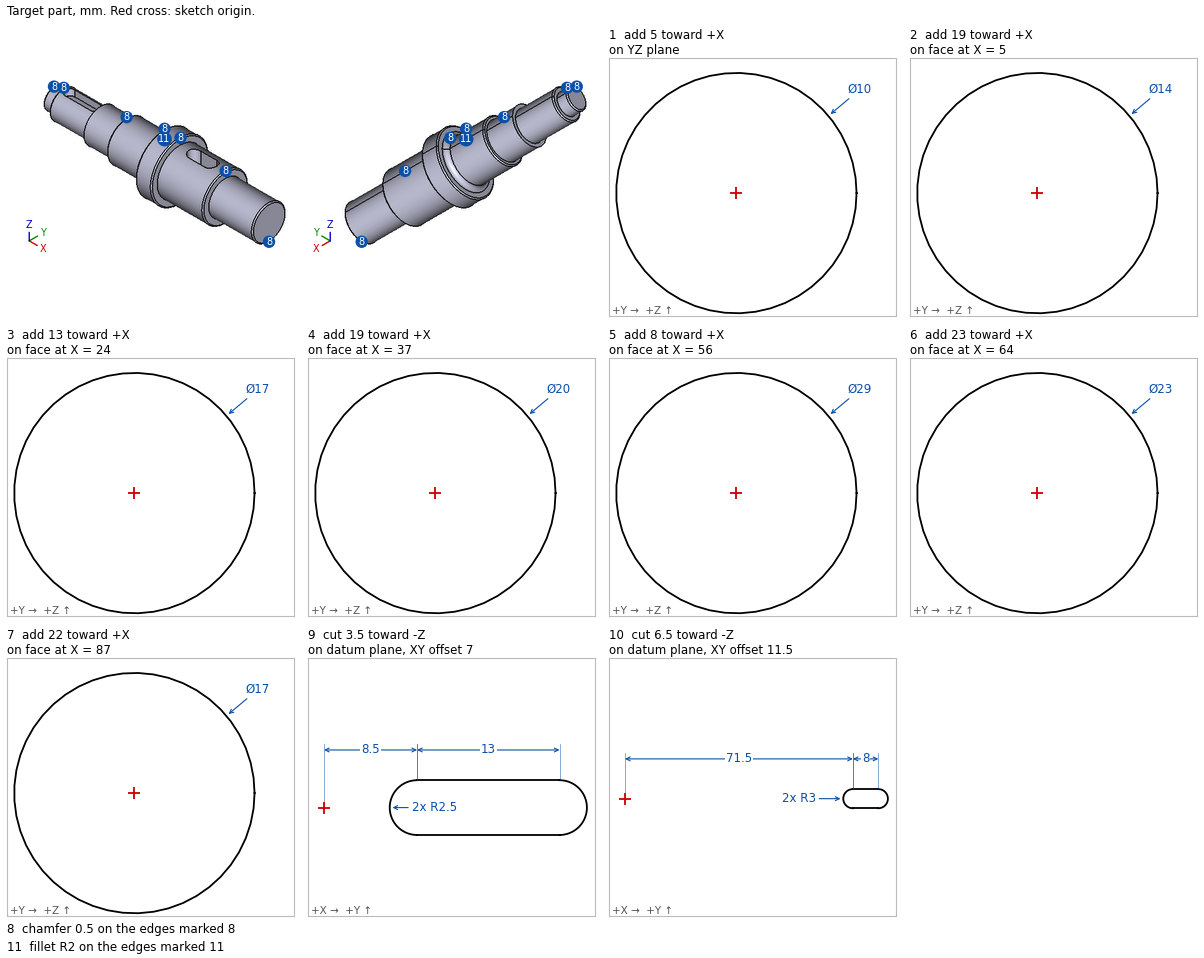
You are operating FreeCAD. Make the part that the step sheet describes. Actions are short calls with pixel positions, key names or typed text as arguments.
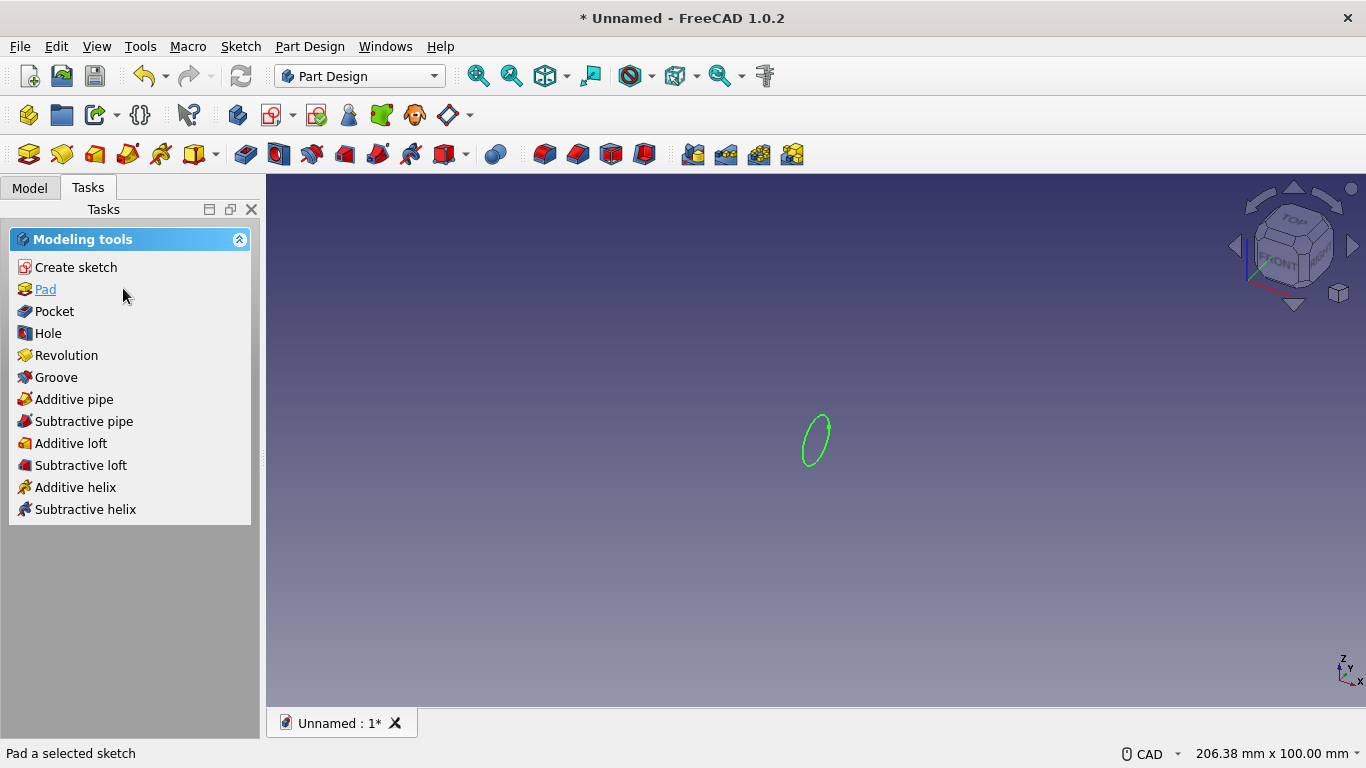
click(29, 154)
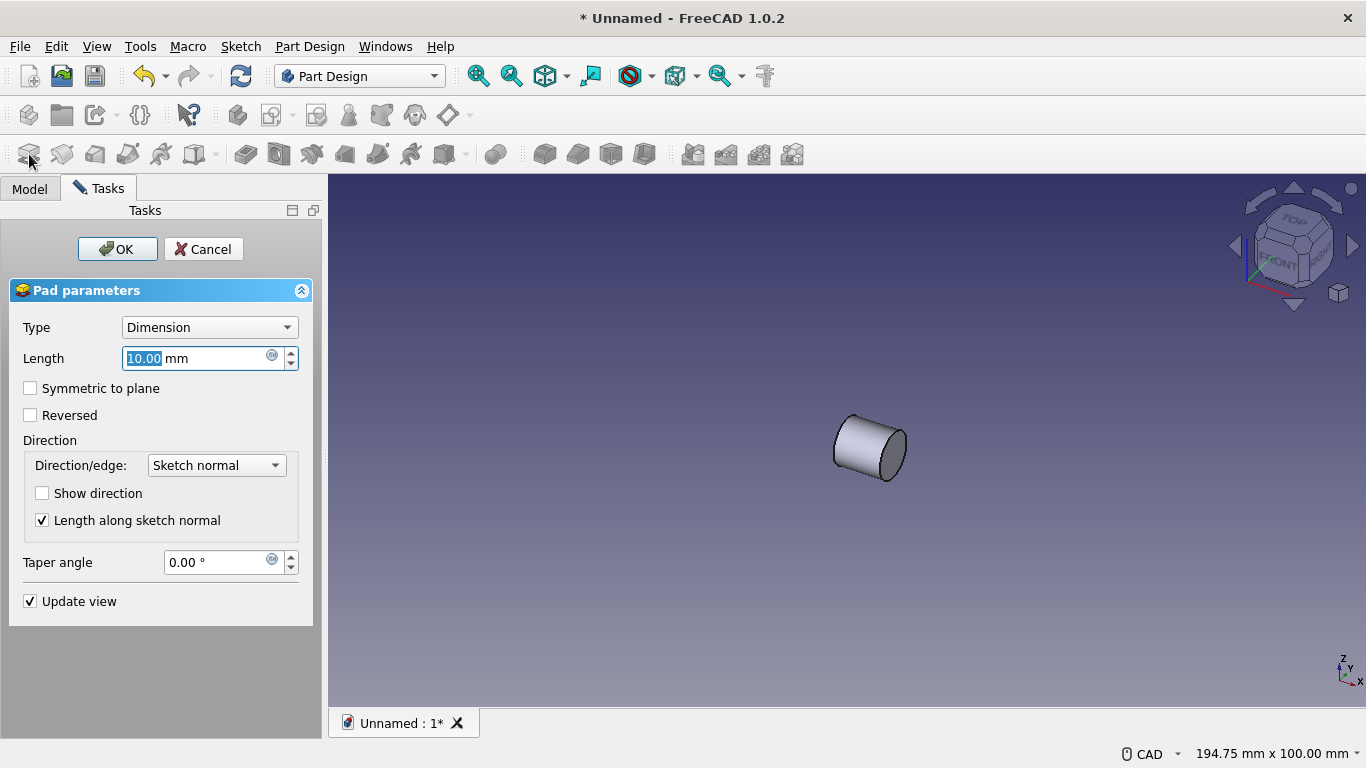
text(5)
key(Tab)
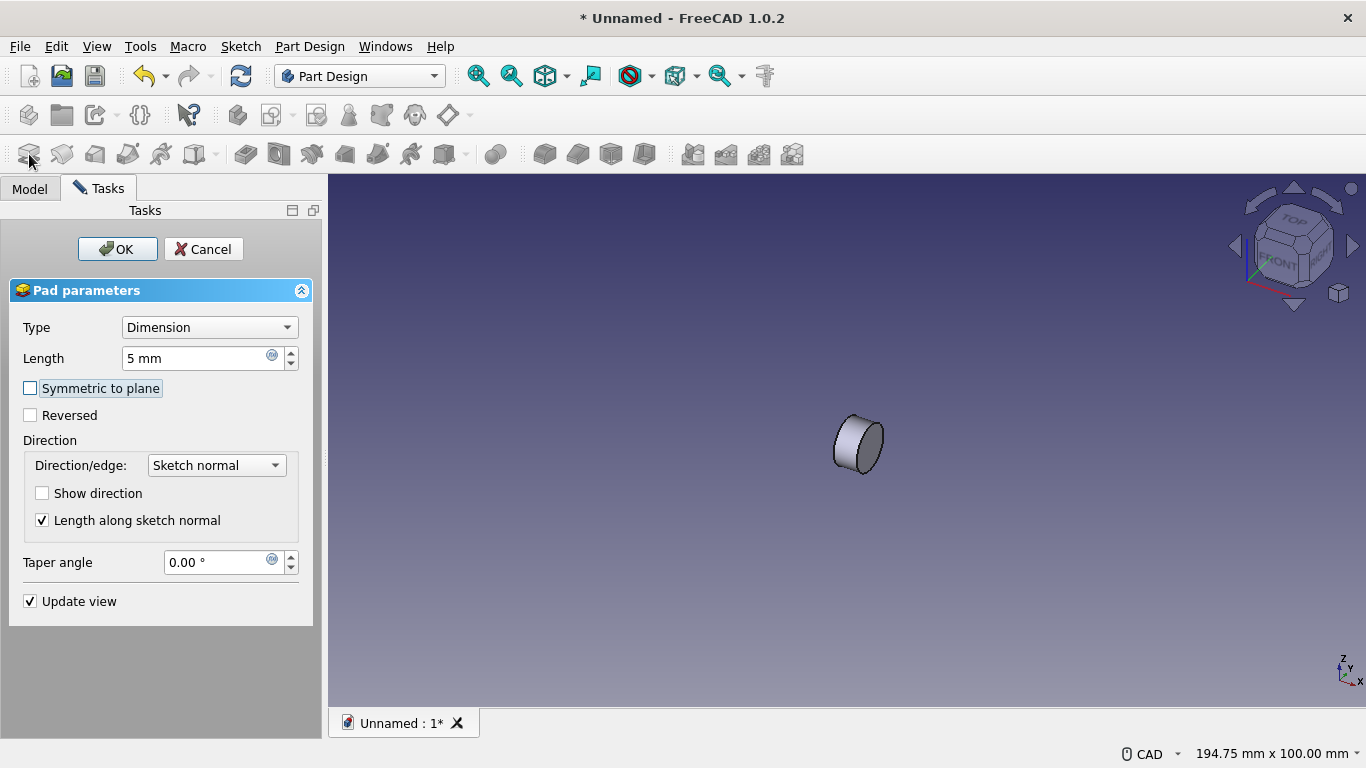
click(118, 249)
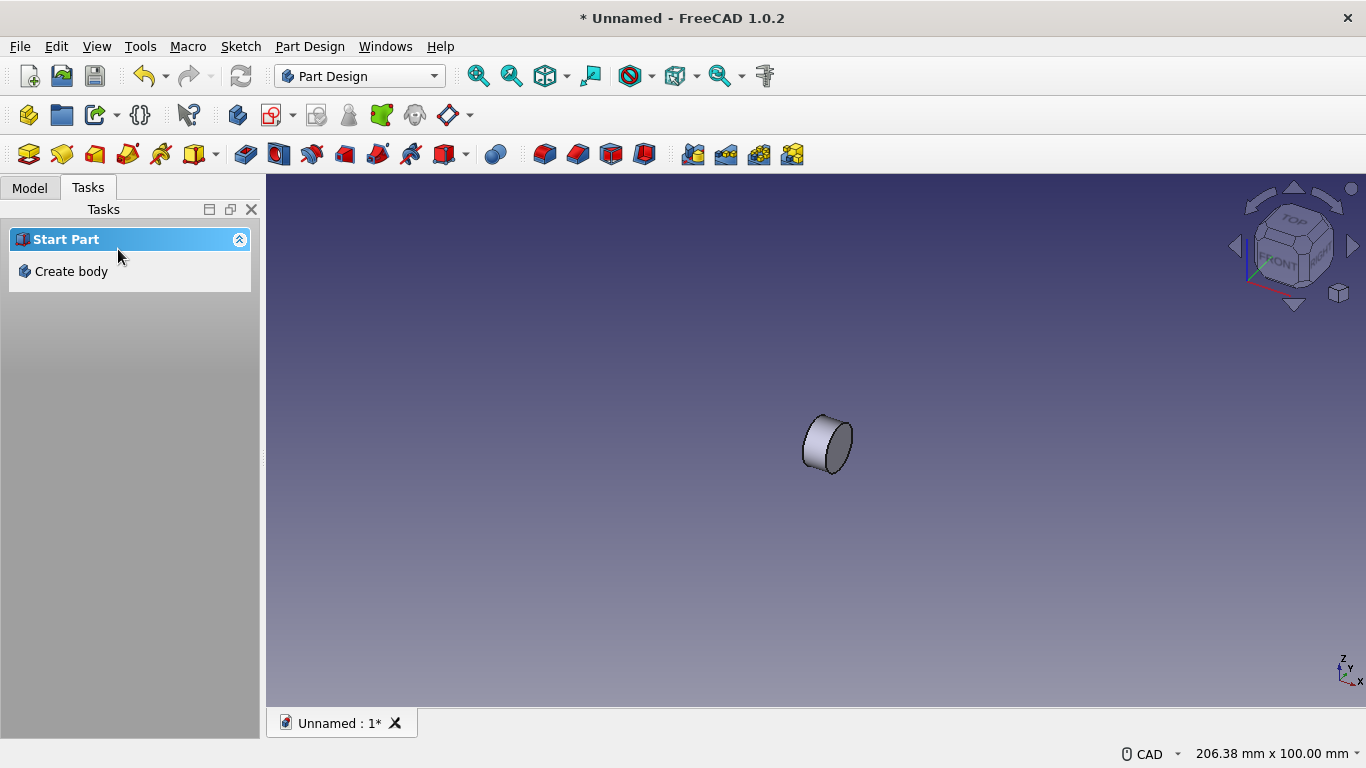
key(v)
key(f)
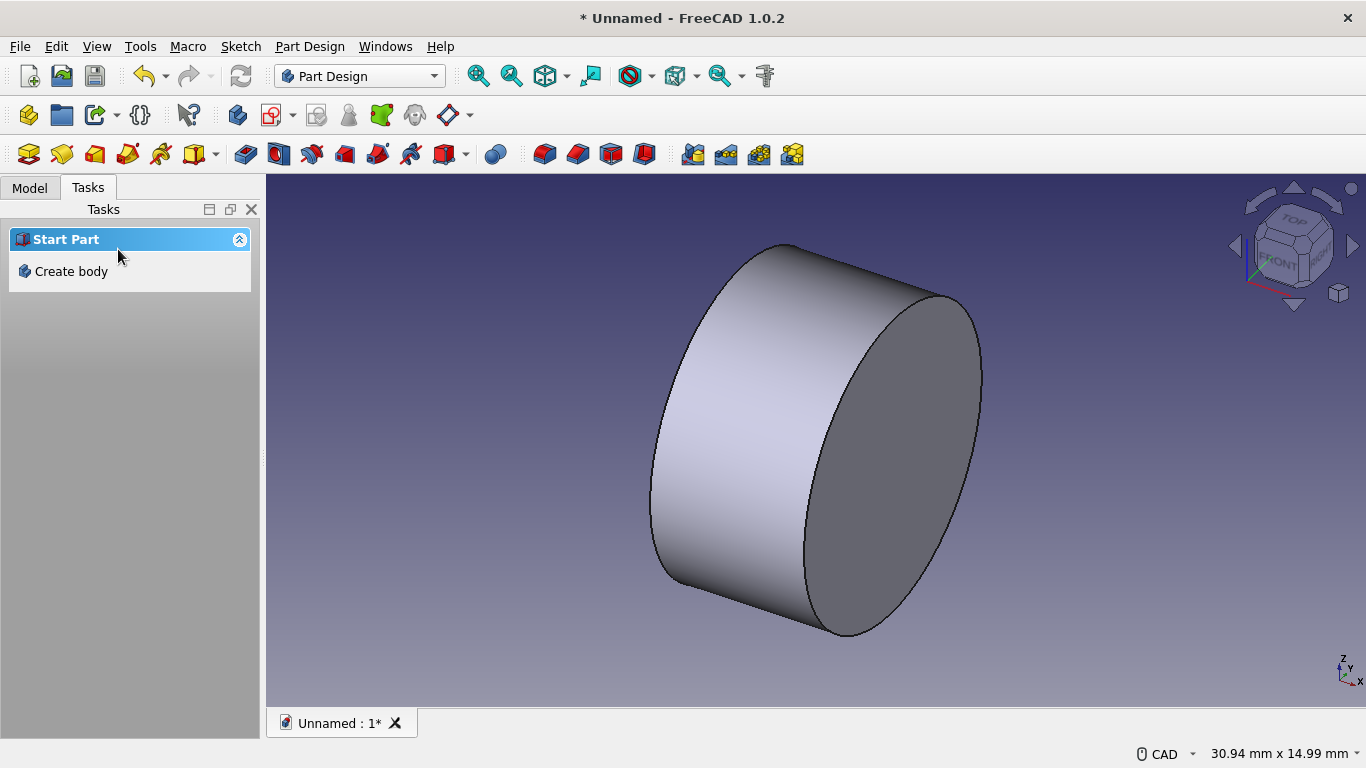
click(893, 465)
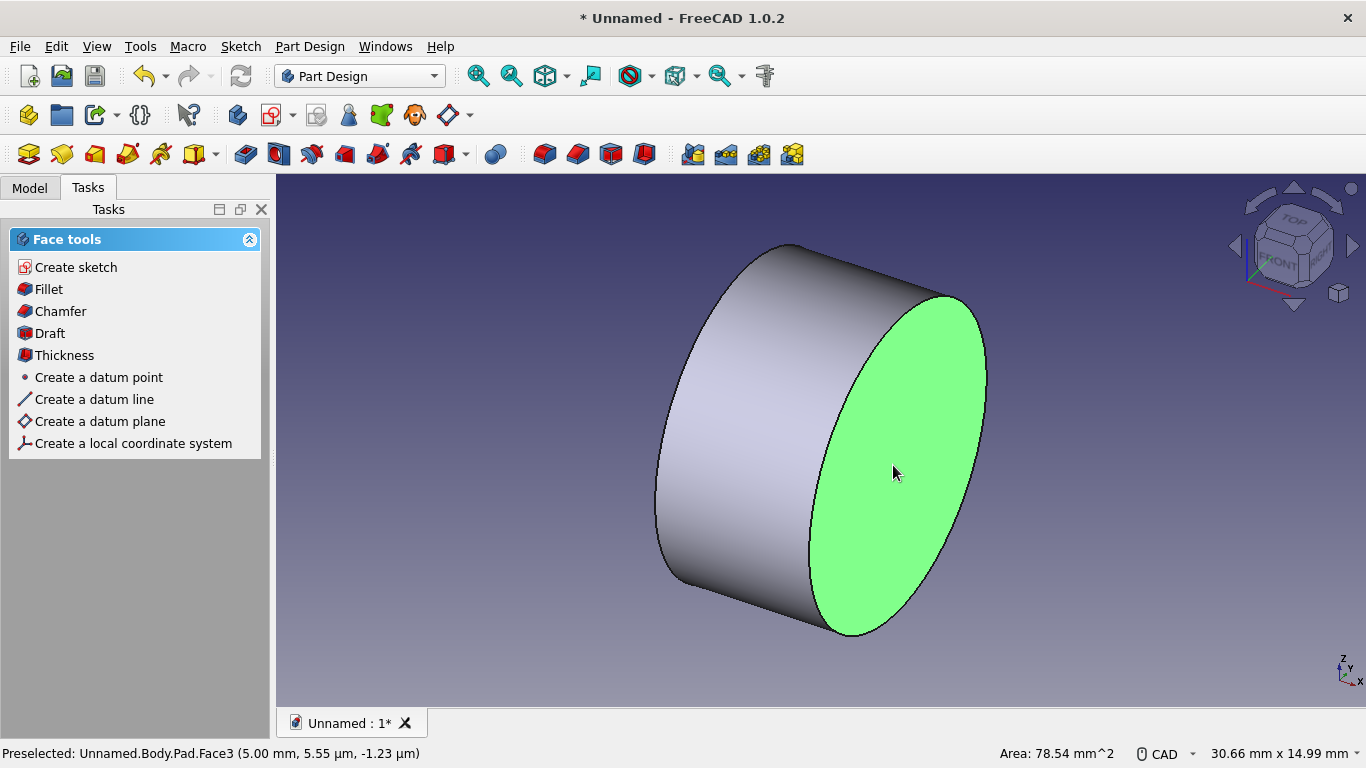
click(270, 116)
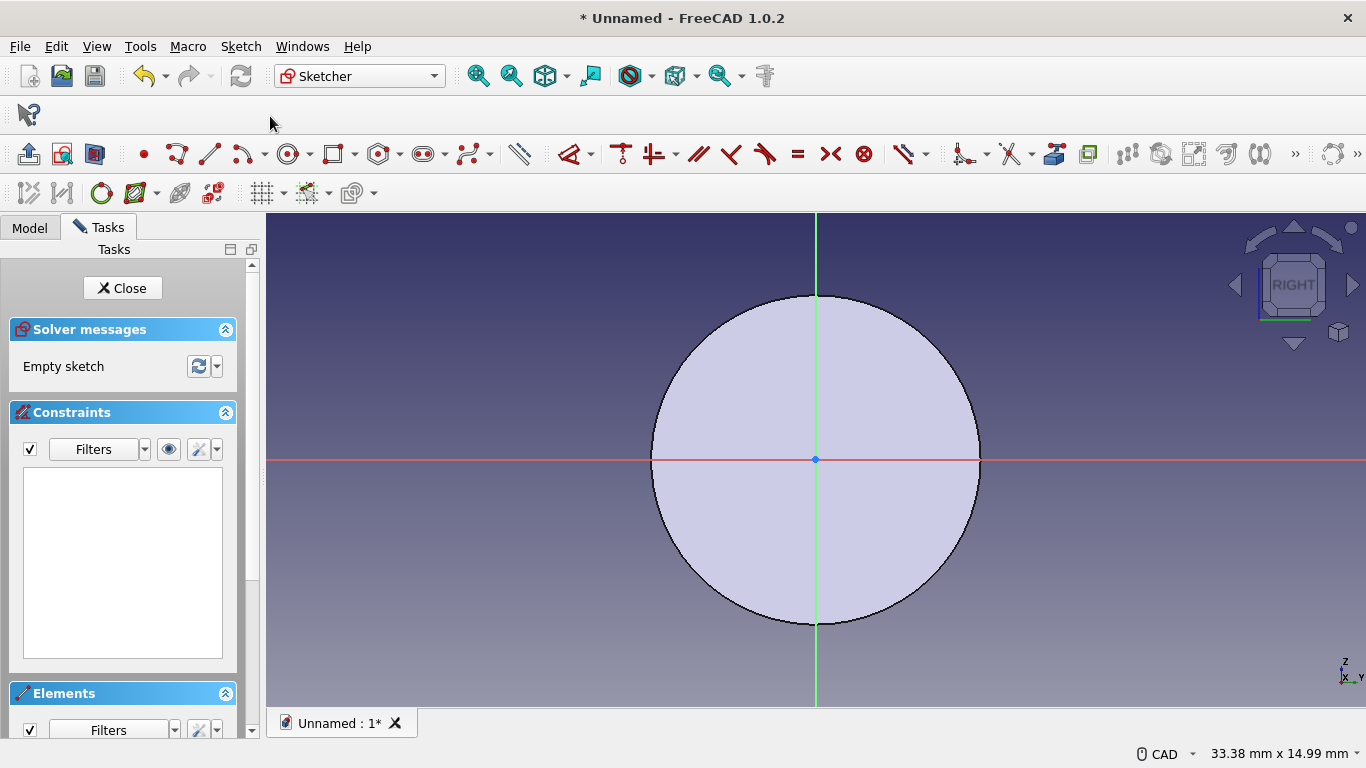
scroll(608, 460, down, 2)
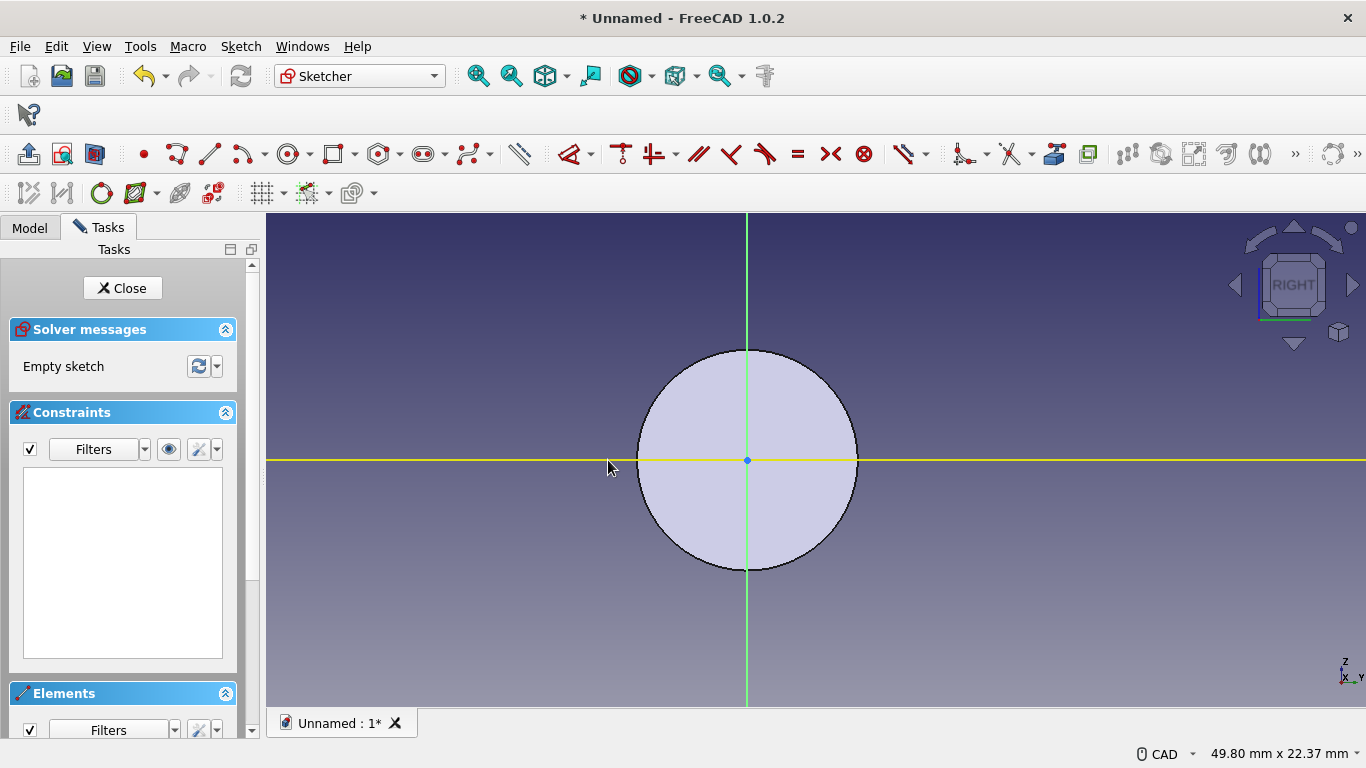
click(288, 154)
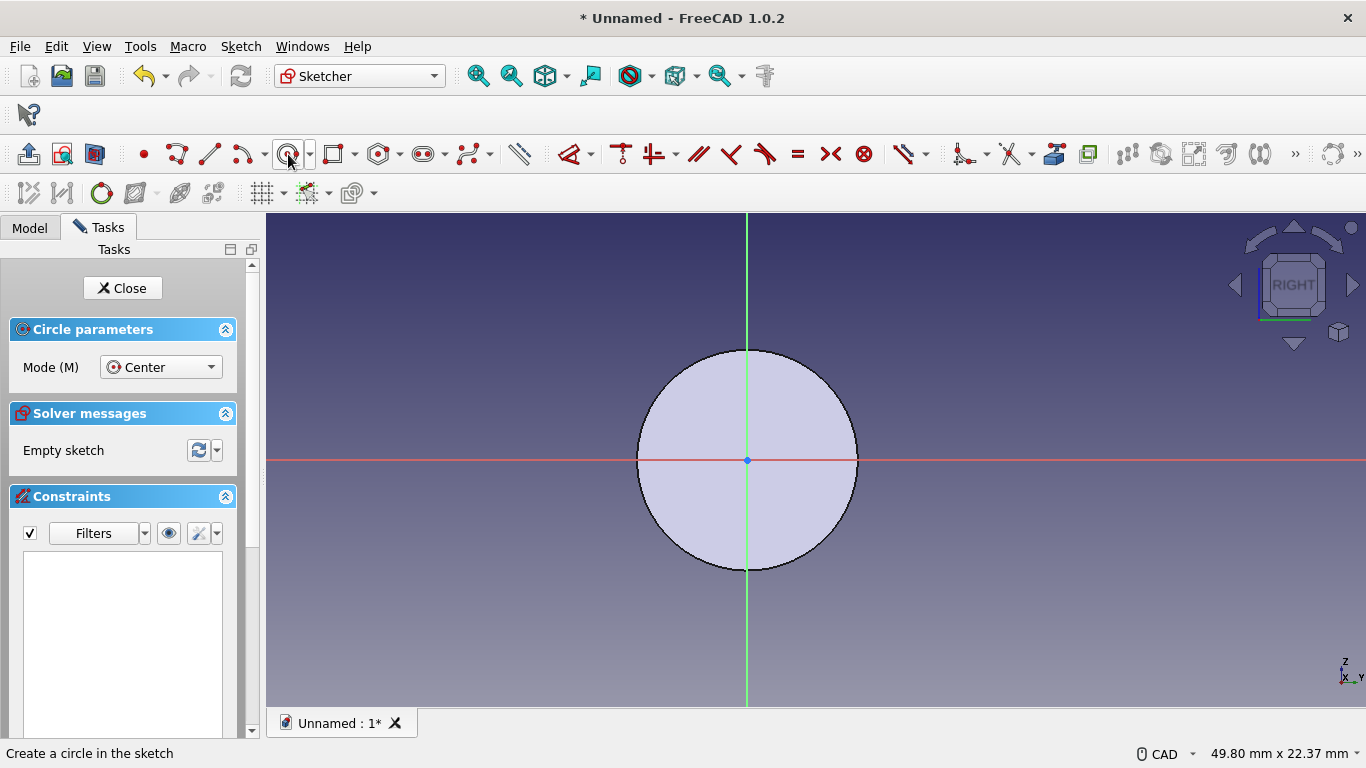
click(747, 460)
move(857, 351)